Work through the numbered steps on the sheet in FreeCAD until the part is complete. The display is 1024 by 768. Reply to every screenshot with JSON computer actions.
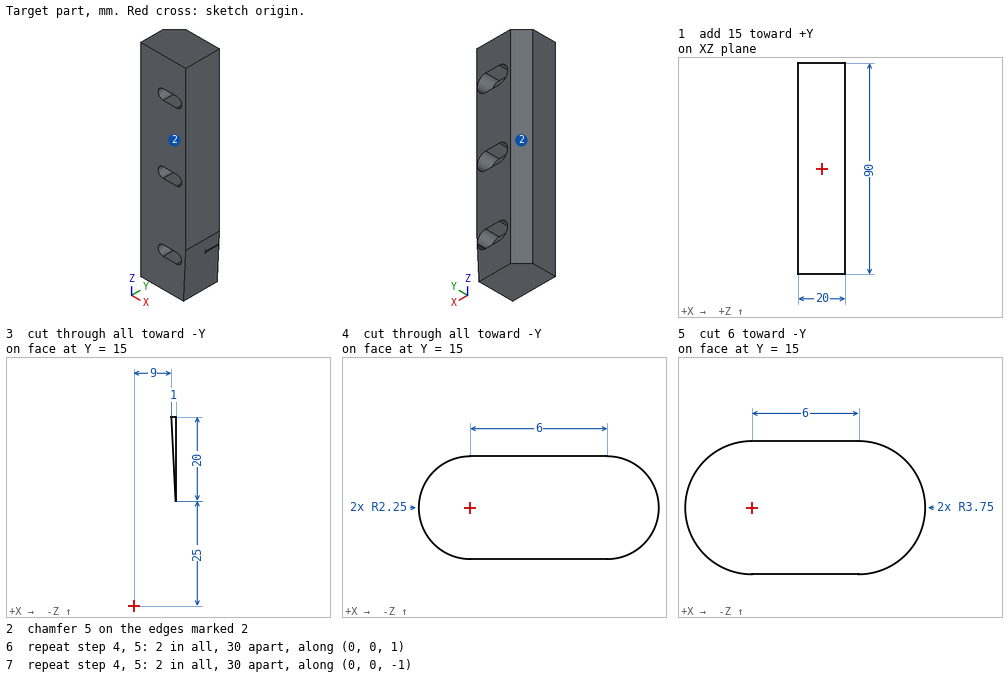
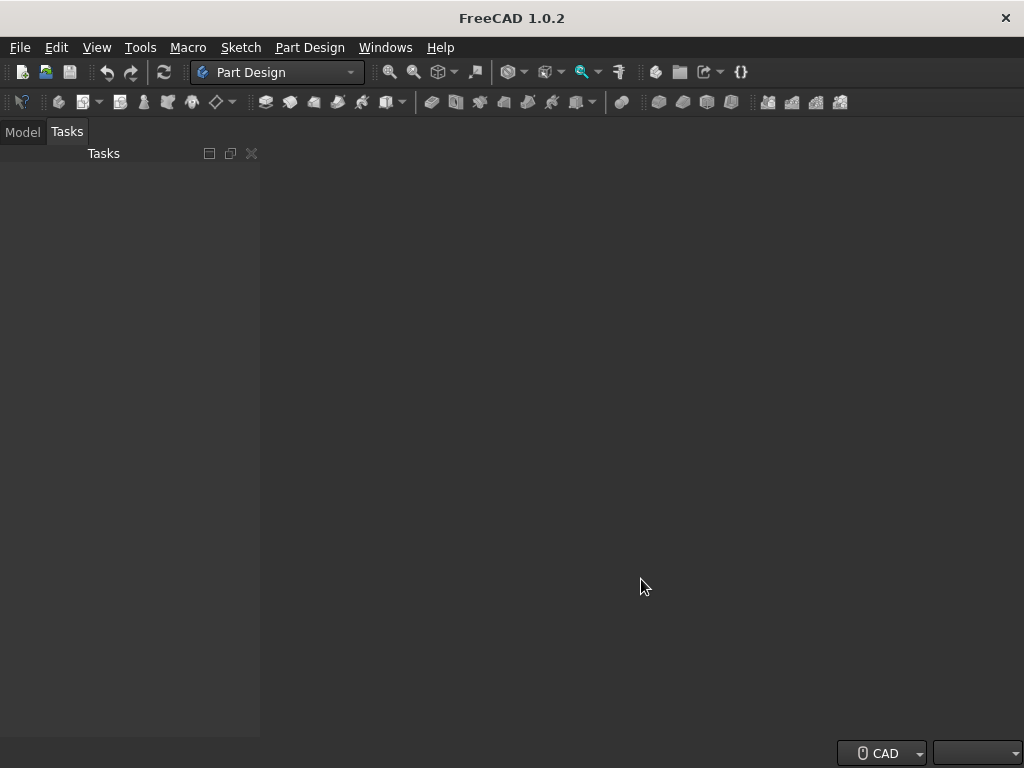
{"action": "left_click", "coordinate": [22, 72]}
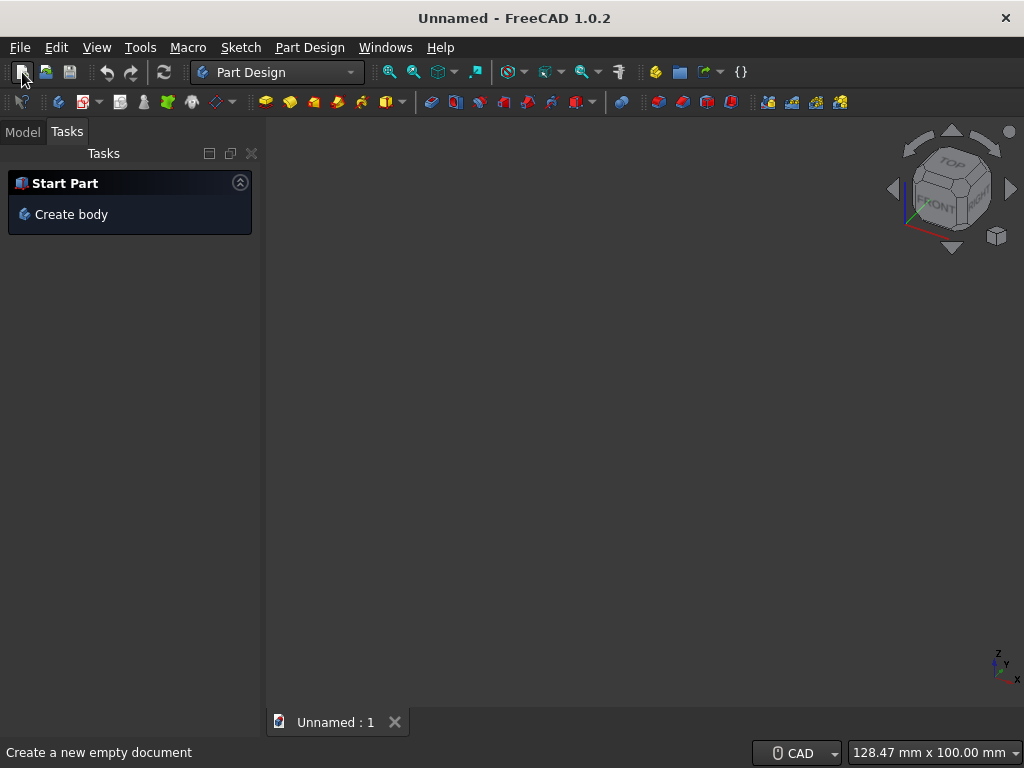
{"action": "left_click", "coordinate": [84, 102]}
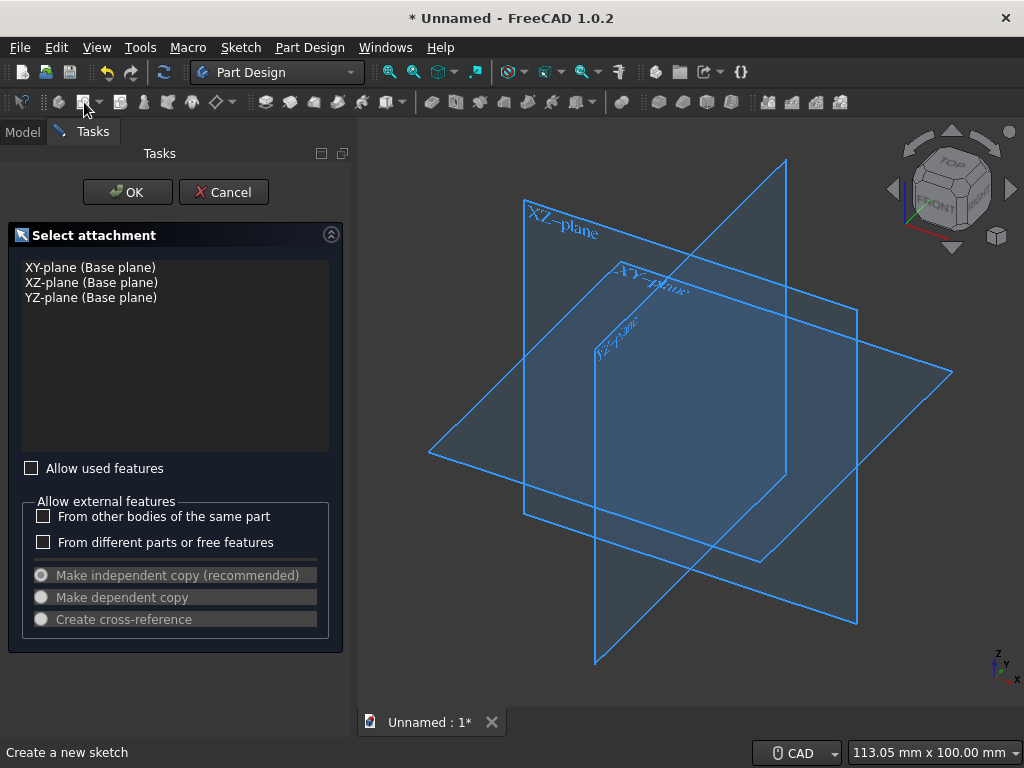
{"action": "left_click", "coordinate": [82, 282]}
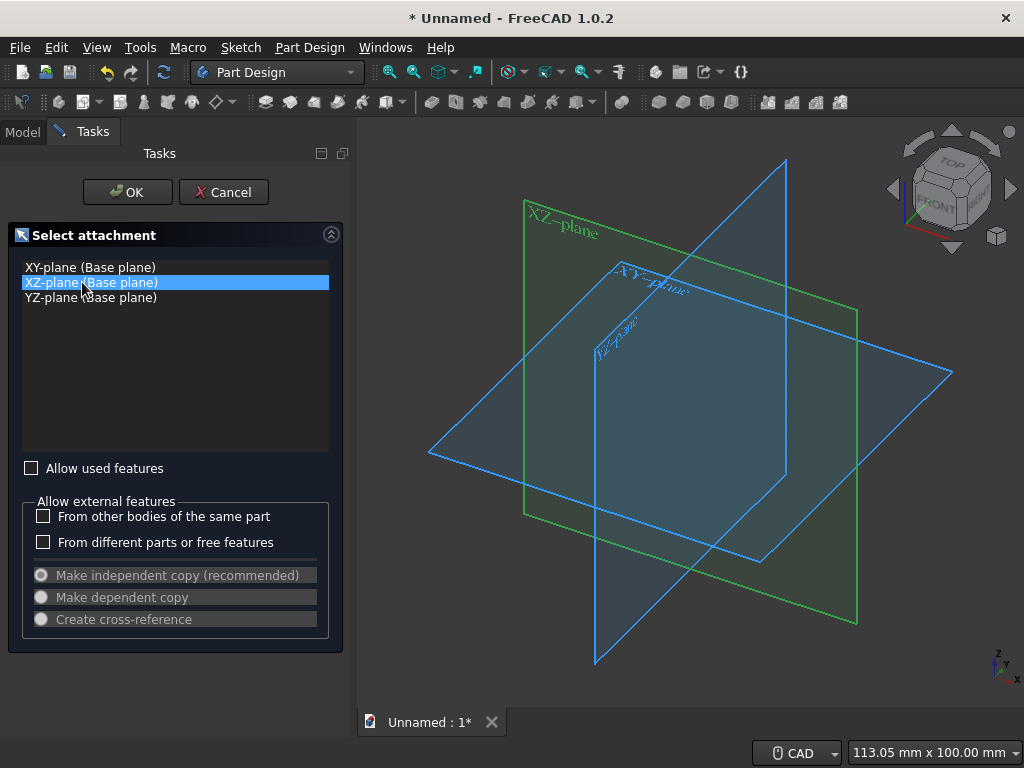
{"action": "left_click", "coordinate": [128, 192]}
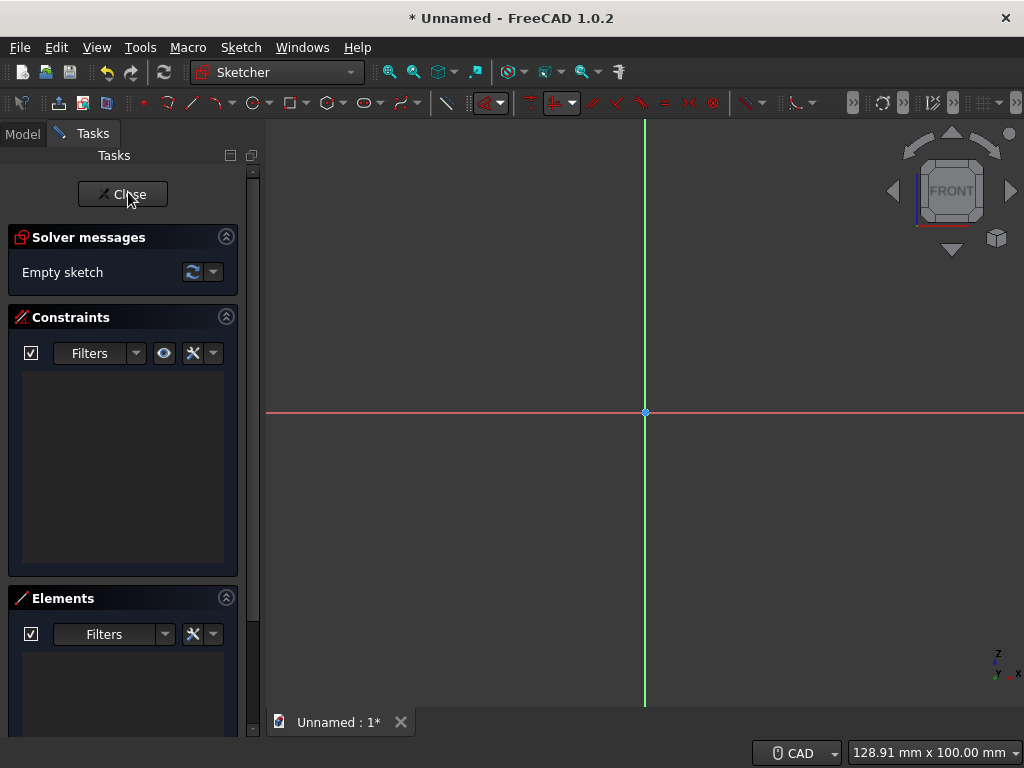
{"action": "scroll", "coordinate": [437, 413], "scroll_direction": "down", "scroll_amount": 2}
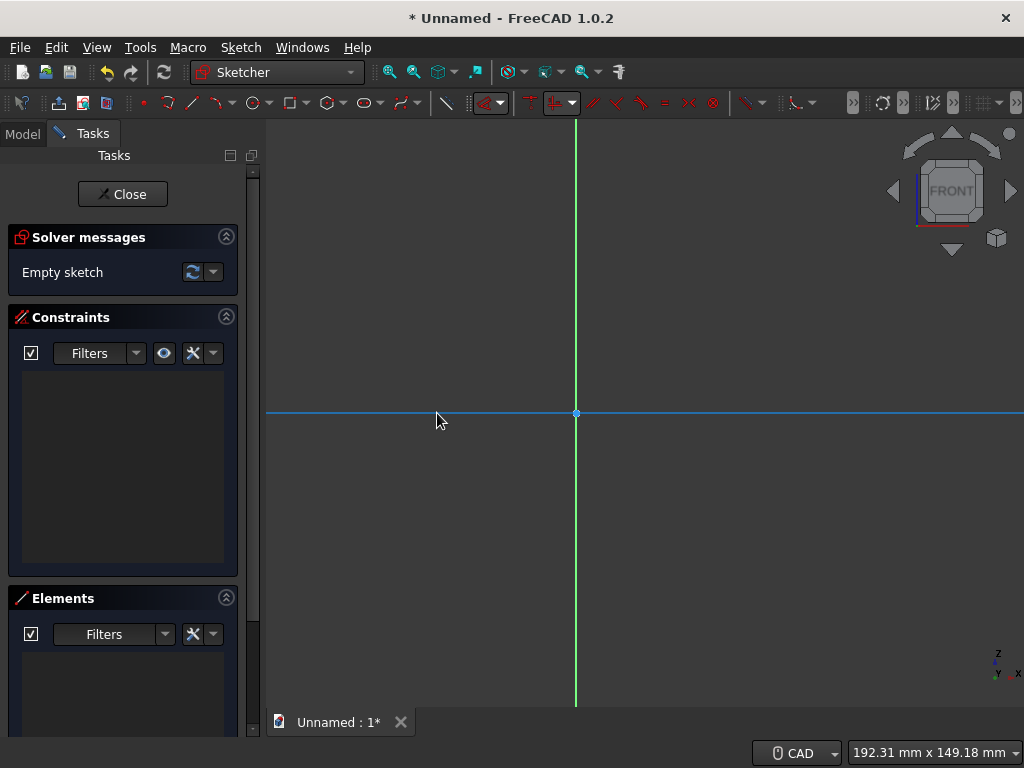
{"action": "key", "text": "g v"}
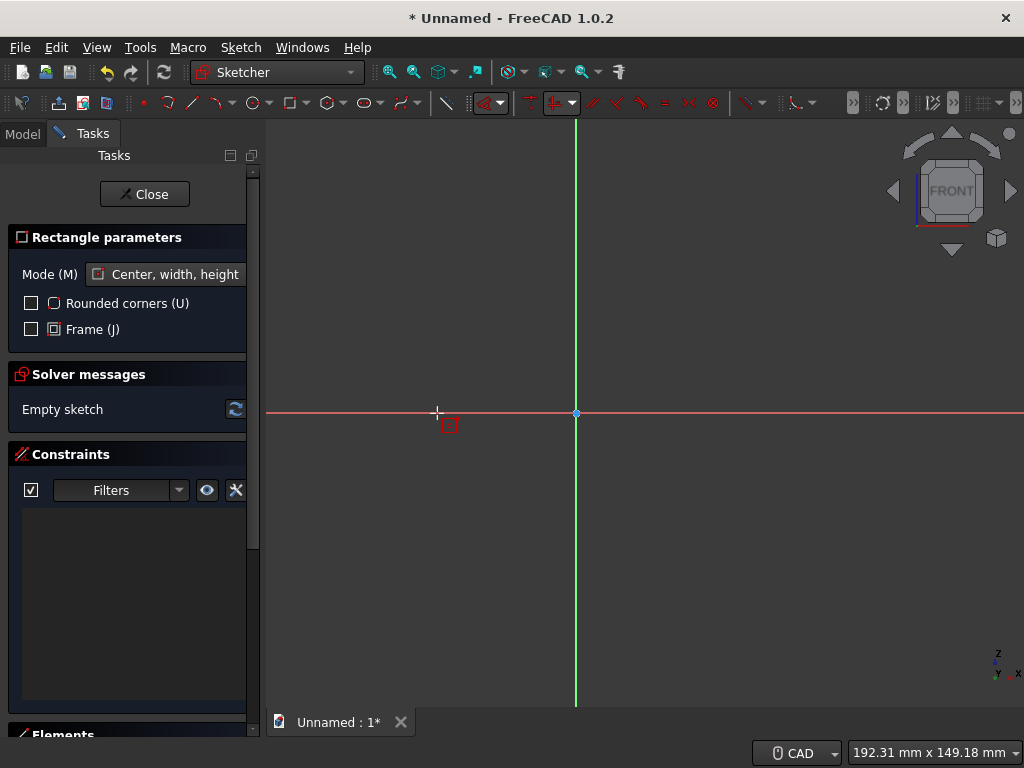
{"action": "left_click", "coordinate": [577, 413]}
{"action": "mouse_move", "coordinate": [616, 236]}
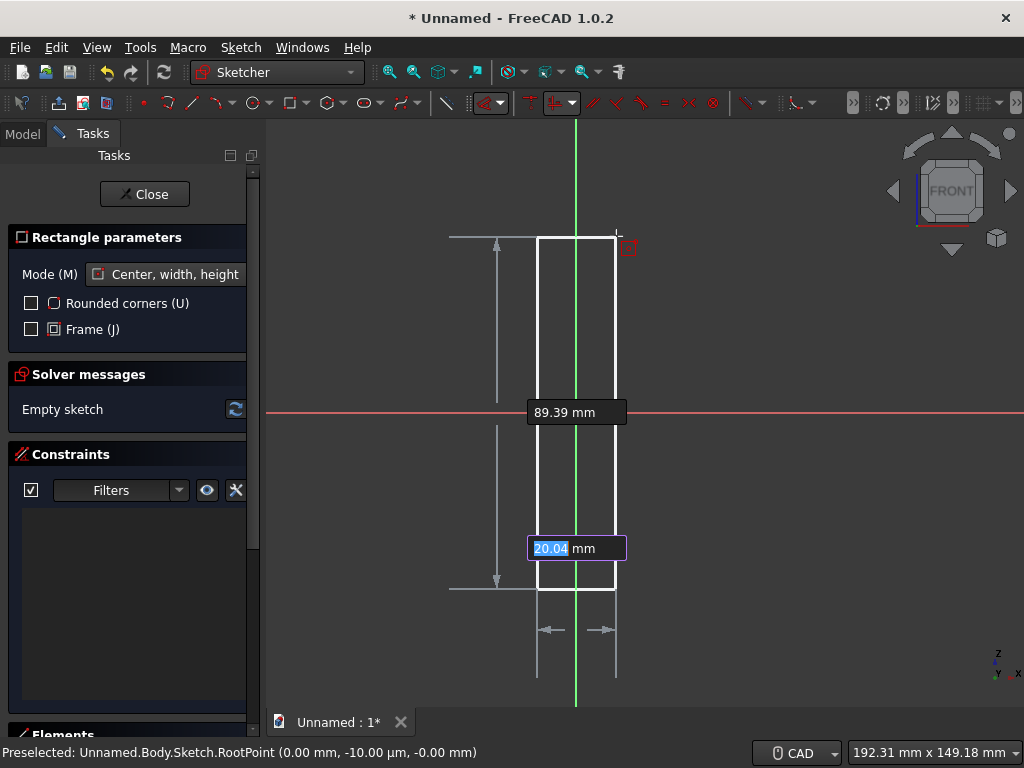
{"action": "type", "text": "20"}
{"action": "key", "text": "Tab"}
{"action": "type", "text": "90"}
{"action": "key", "text": "Return"}
{"action": "key", "text": "Escape"}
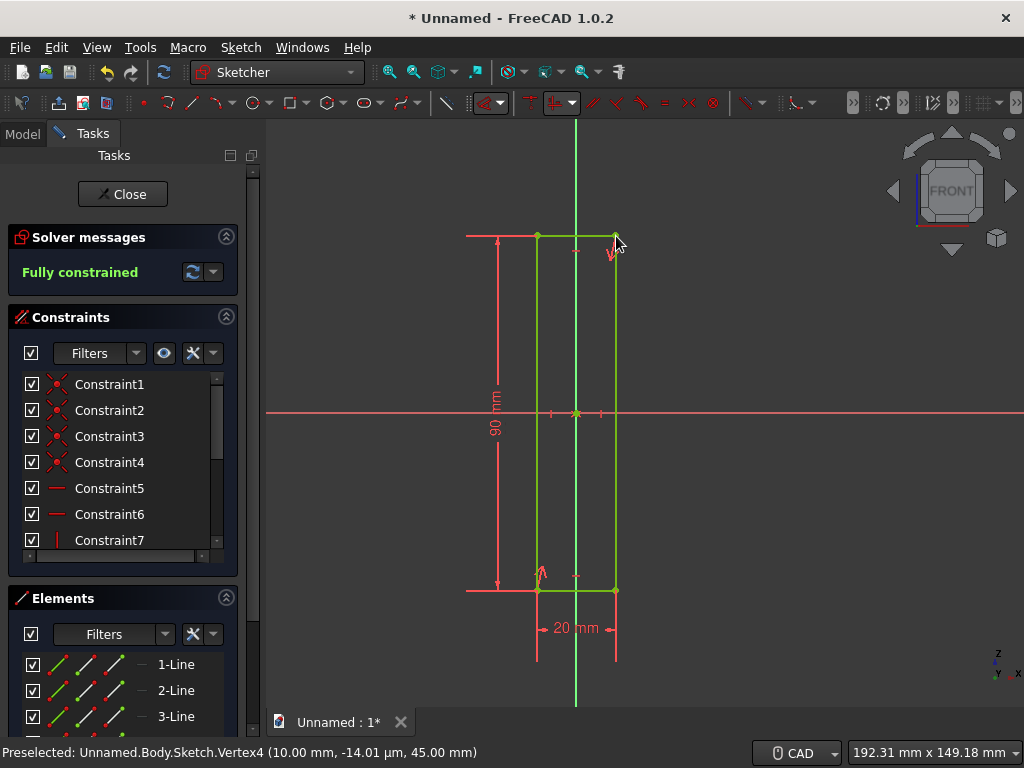
{"action": "left_click", "coordinate": [123, 194]}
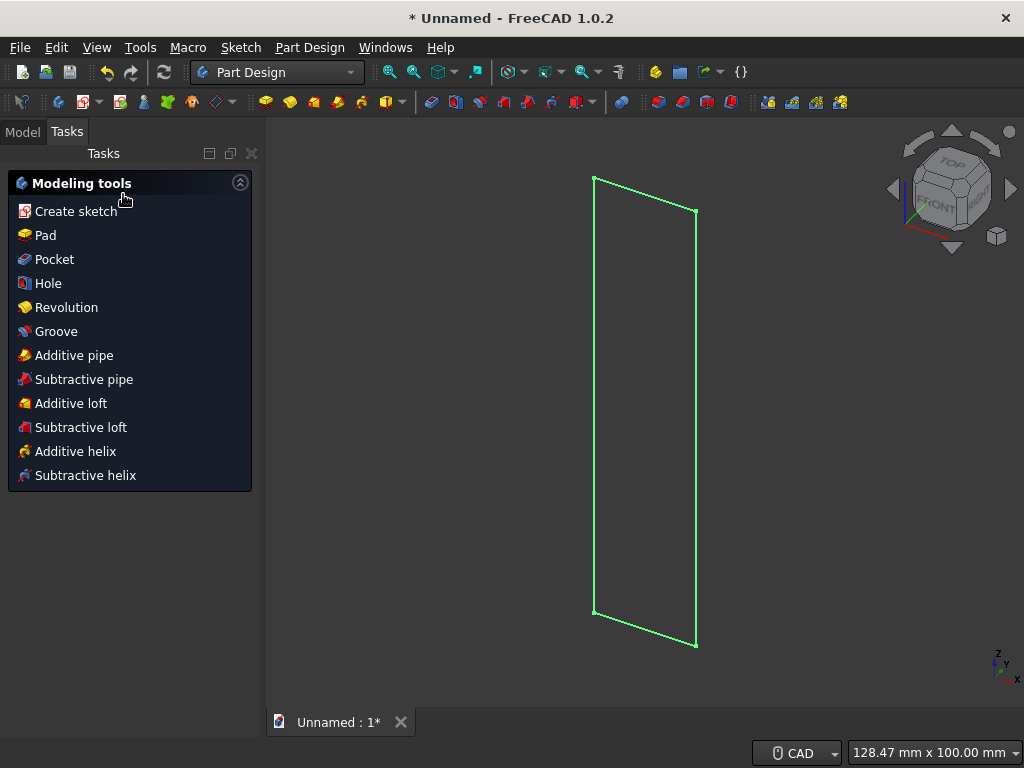
{"action": "left_click", "coordinate": [266, 102]}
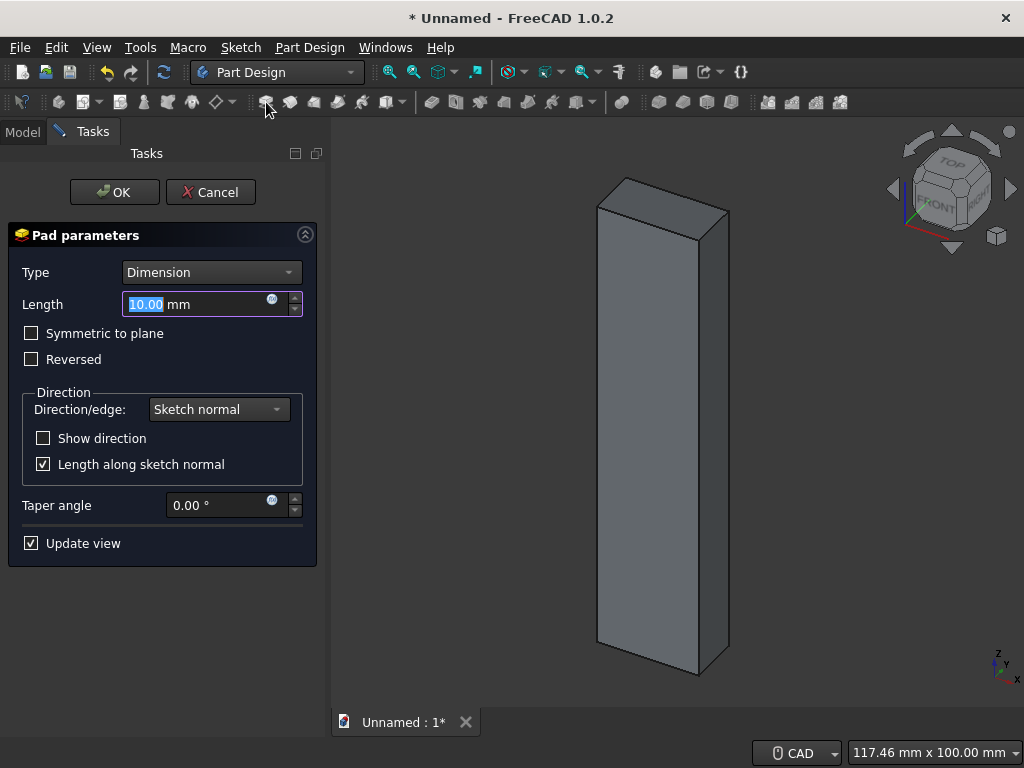
{"action": "type", "text": "15"}
{"action": "key", "text": "Tab"}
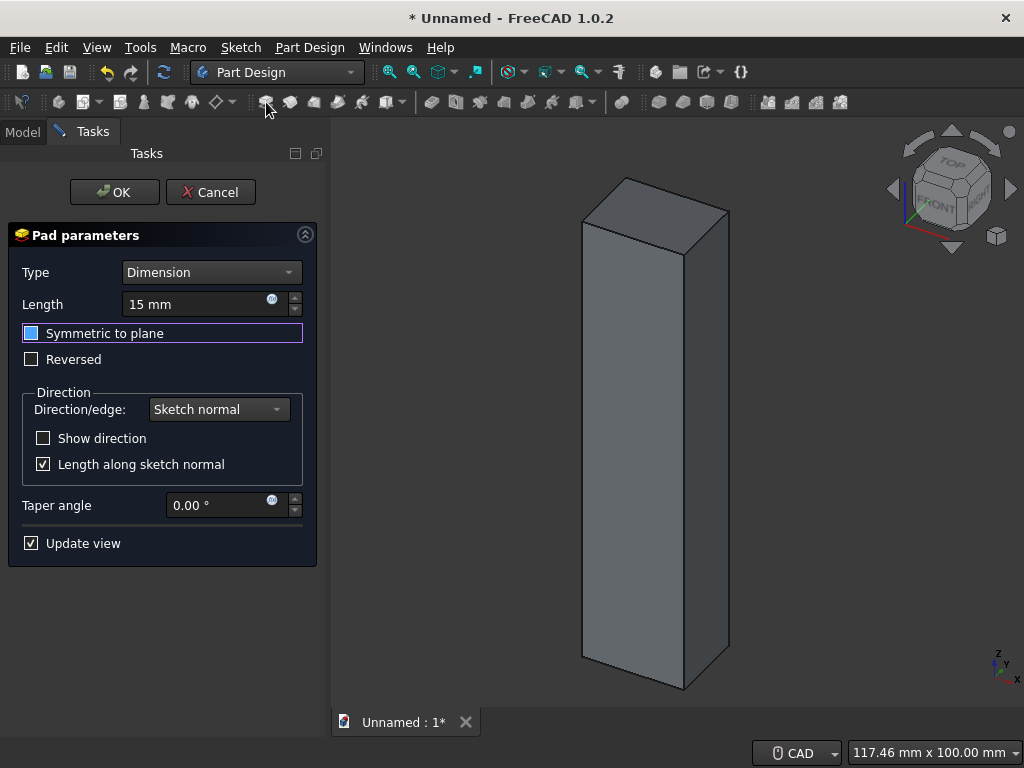
{"action": "left_click", "coordinate": [30, 359]}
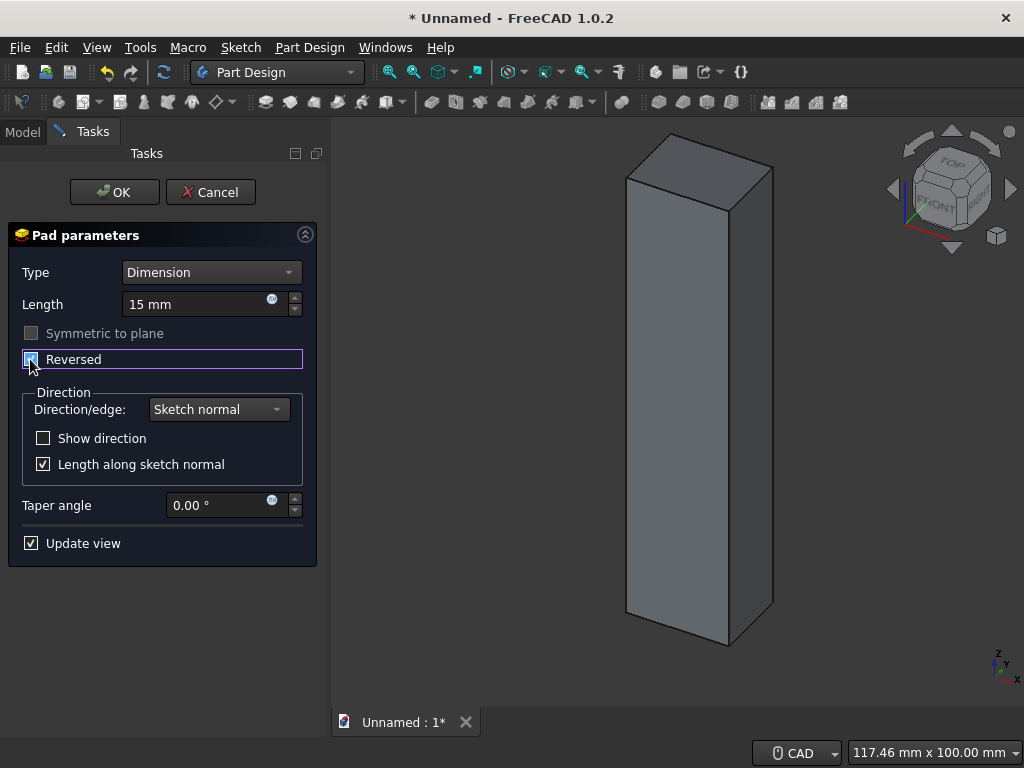
{"action": "left_click", "coordinate": [115, 192]}